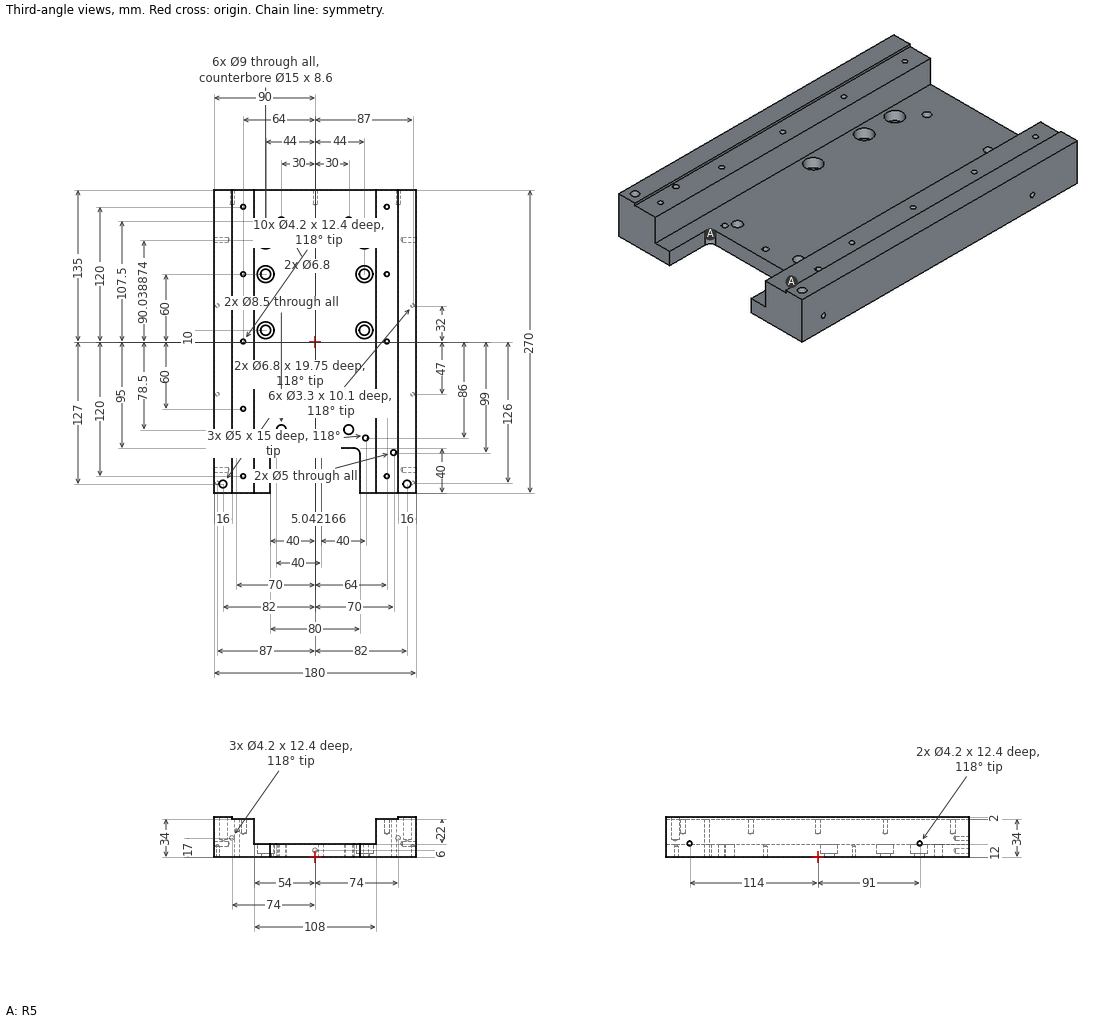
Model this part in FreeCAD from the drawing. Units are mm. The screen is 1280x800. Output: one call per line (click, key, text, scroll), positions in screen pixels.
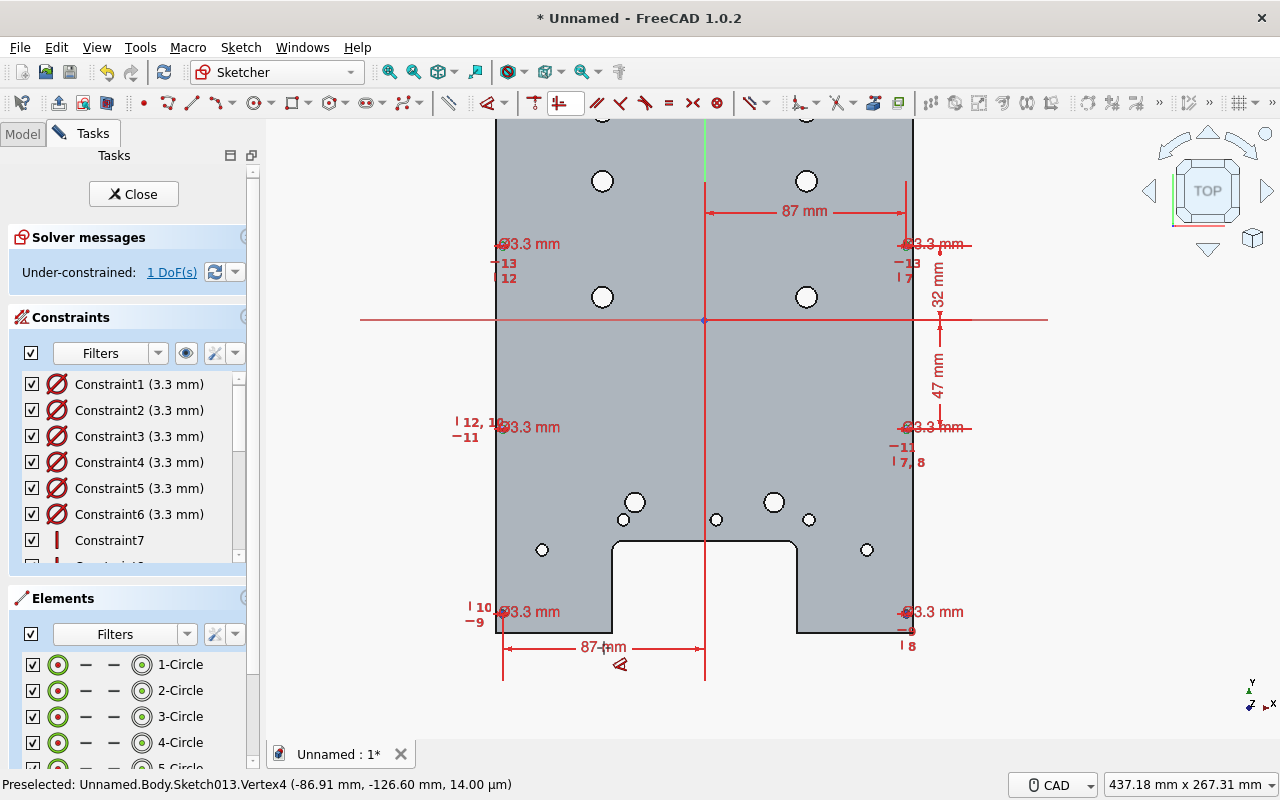
click(906, 614)
click(940, 467)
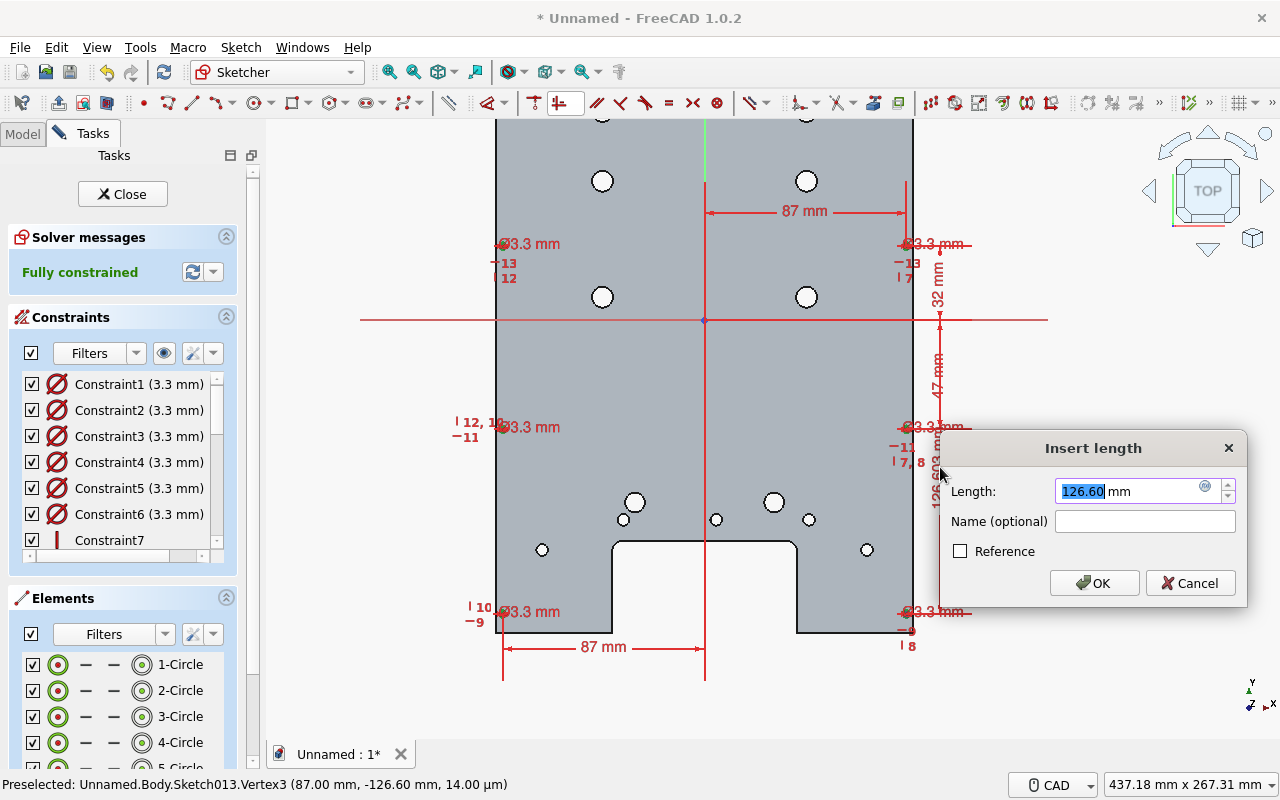
text(126)
key(Return)
key(Escape)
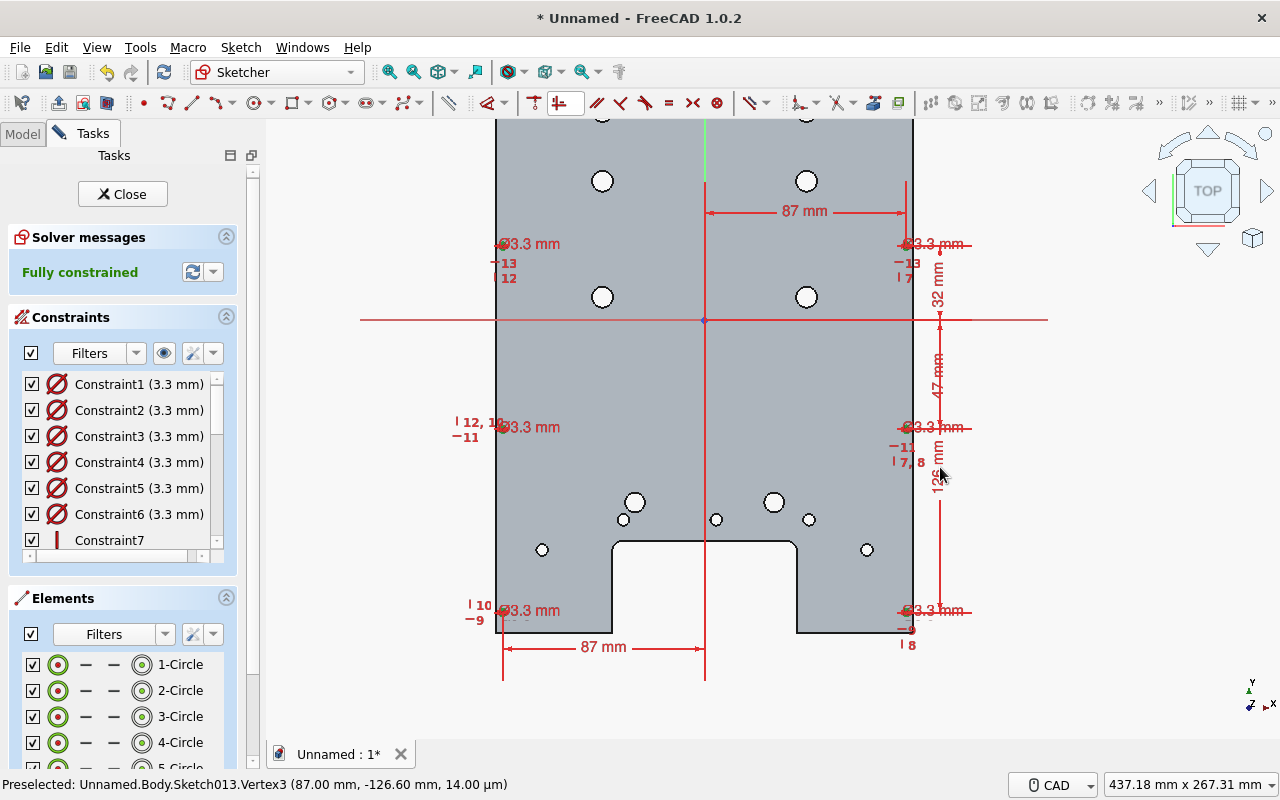
click(123, 194)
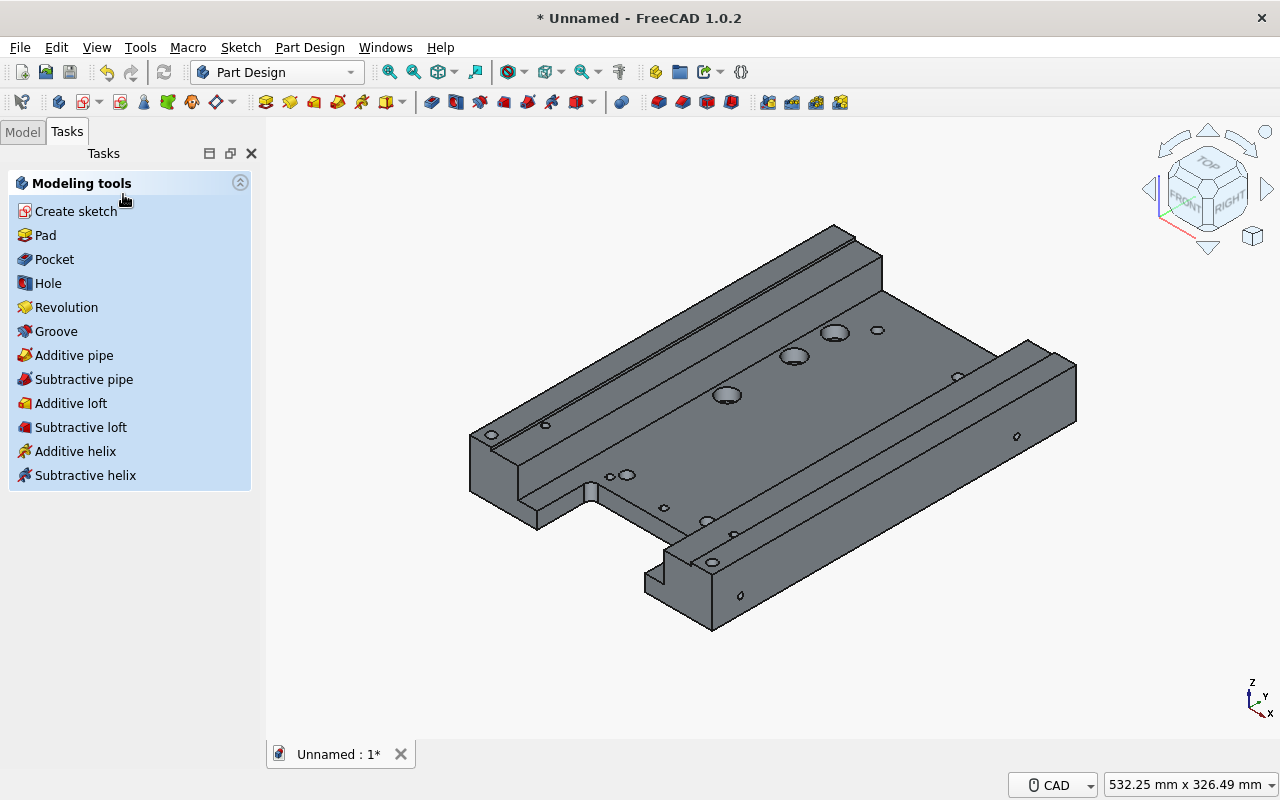
click(456, 102)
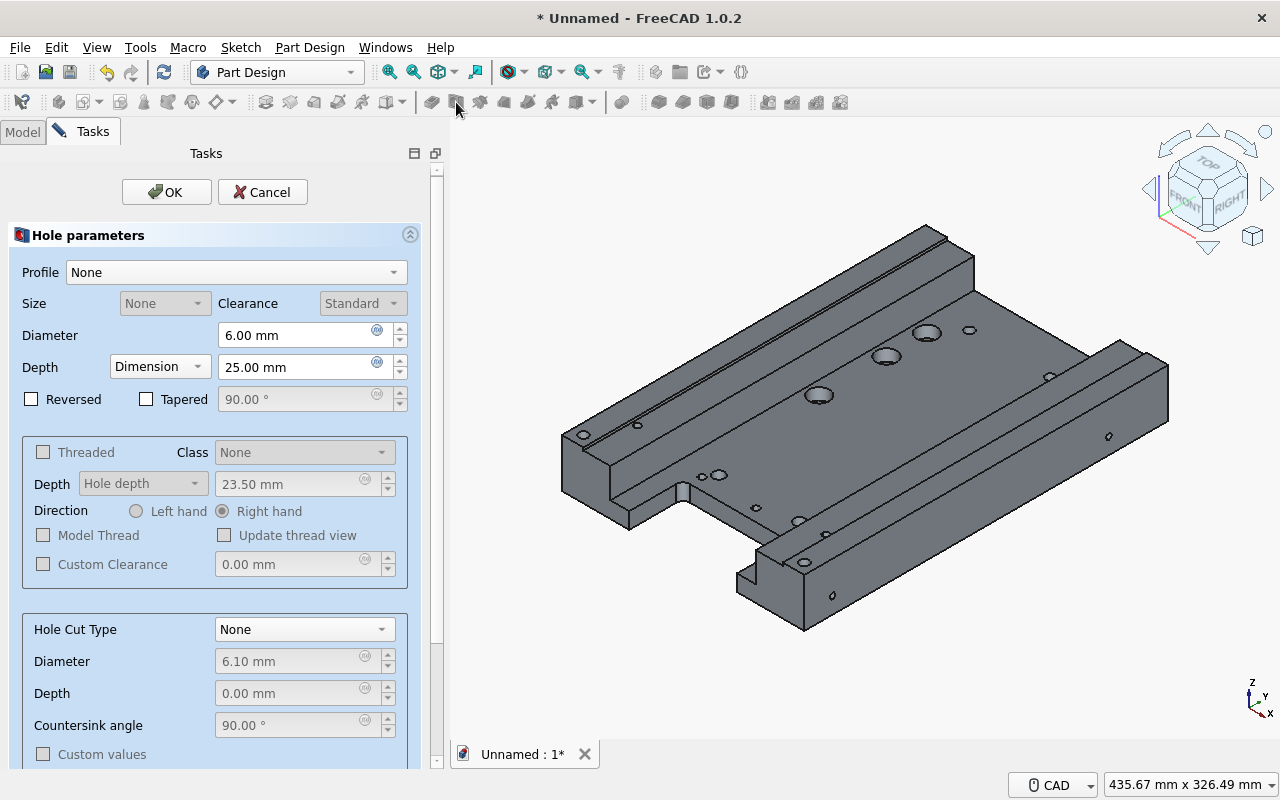
triple_click(305, 335)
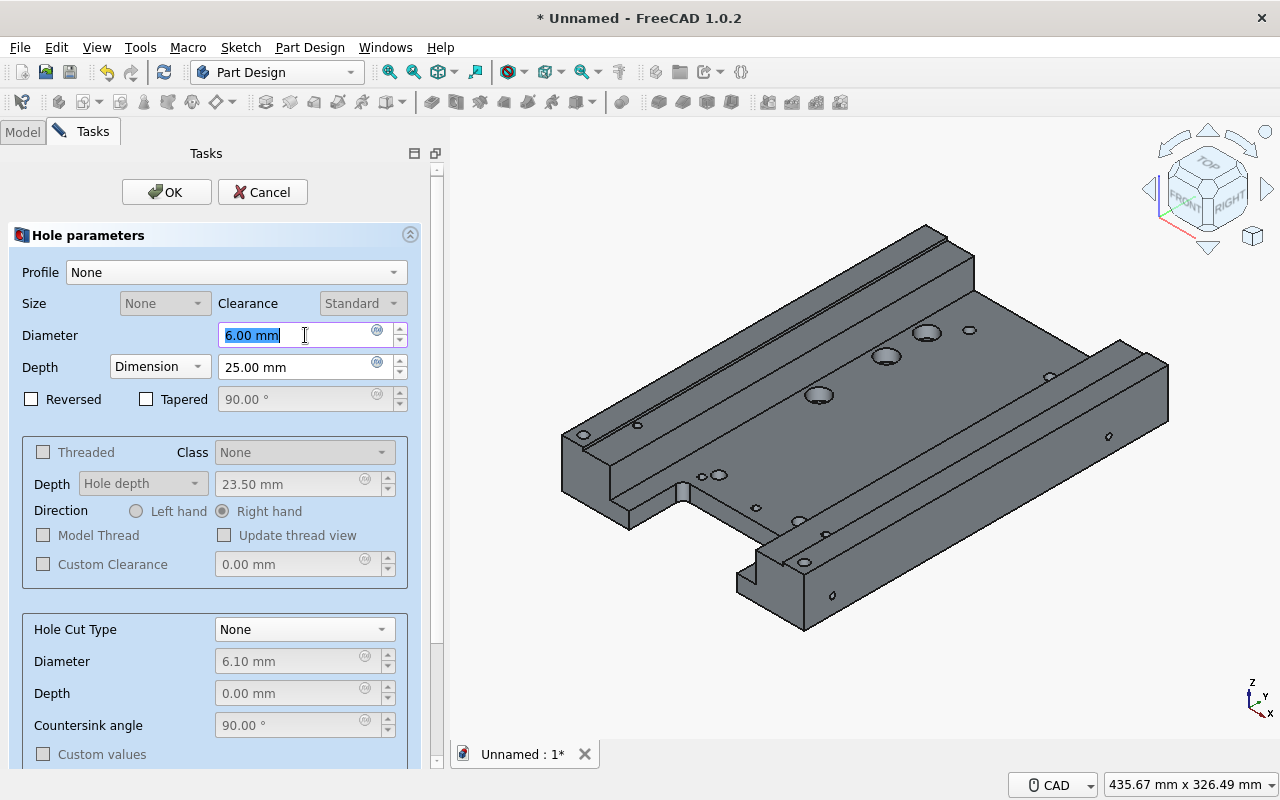
text(3.3)
key(Tab)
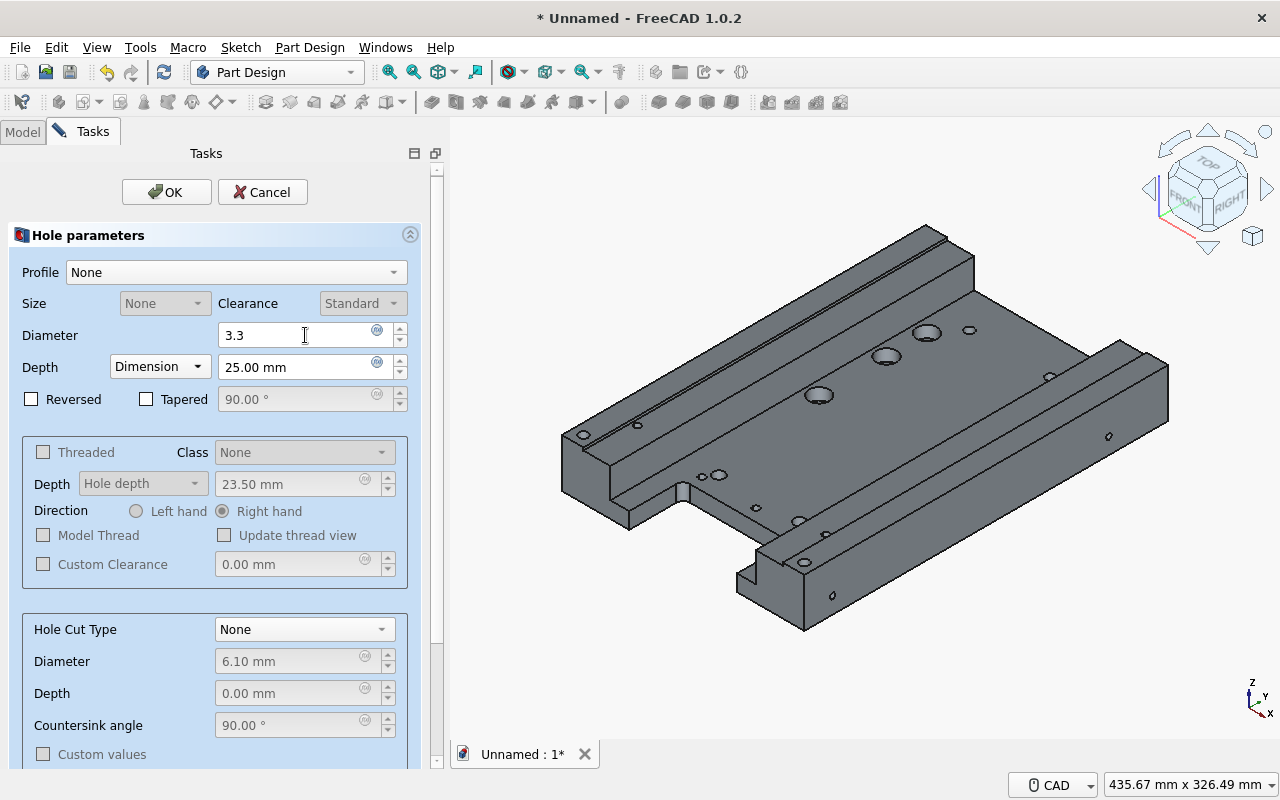
triple_click(305, 367)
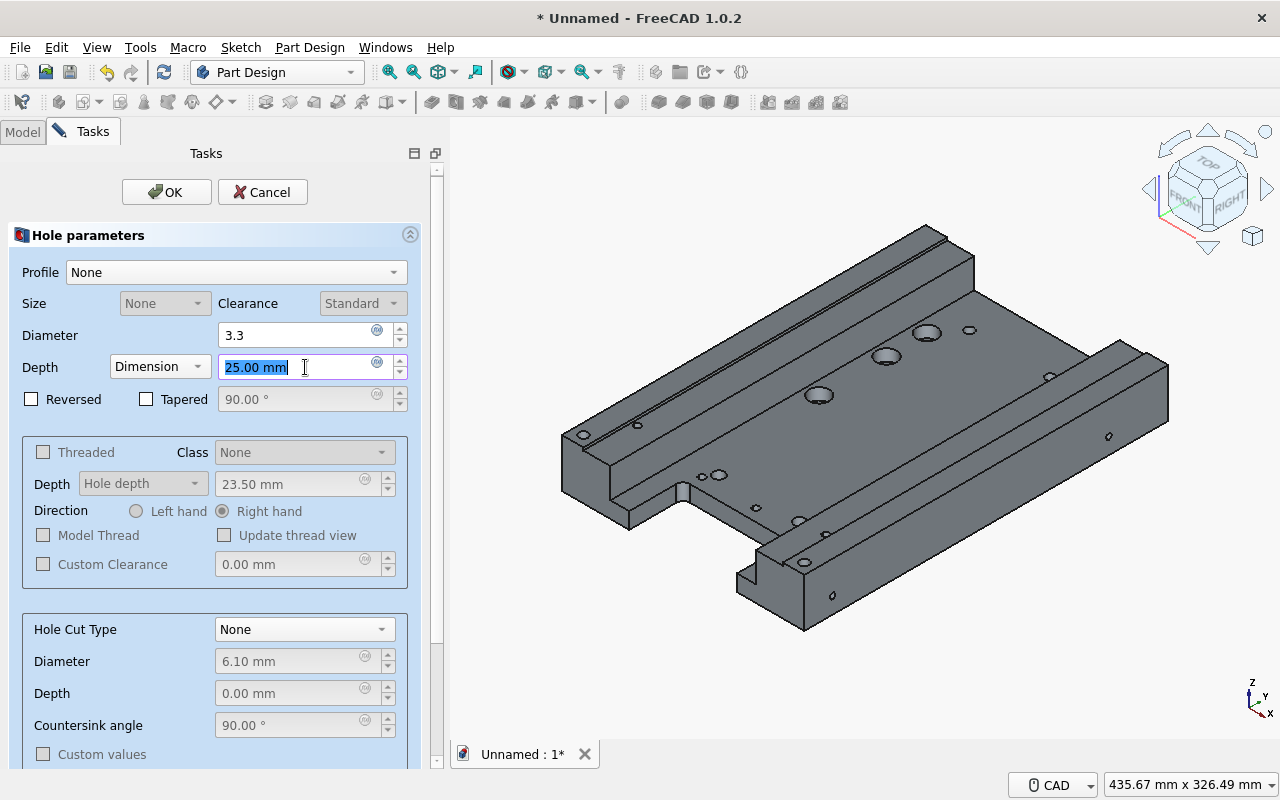
text(10.1)
key(Tab)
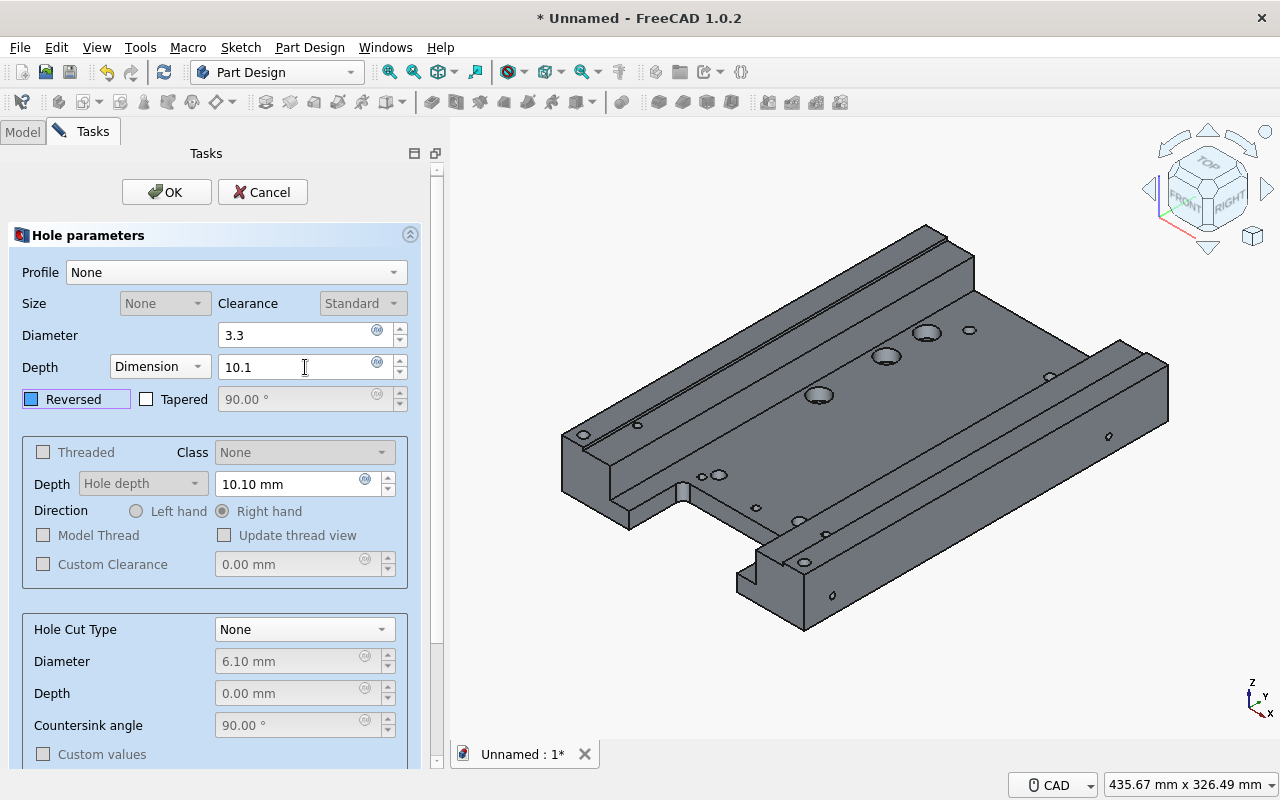
click(30, 399)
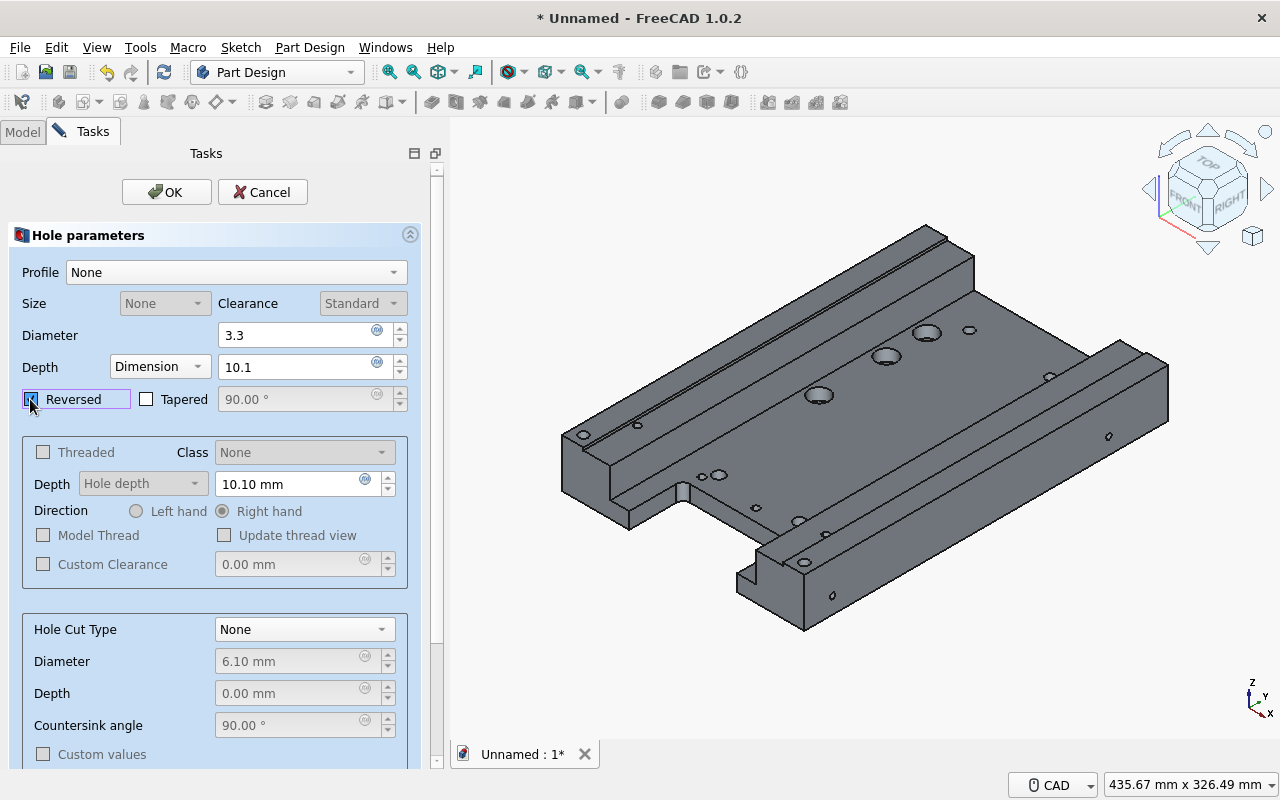
click(167, 192)